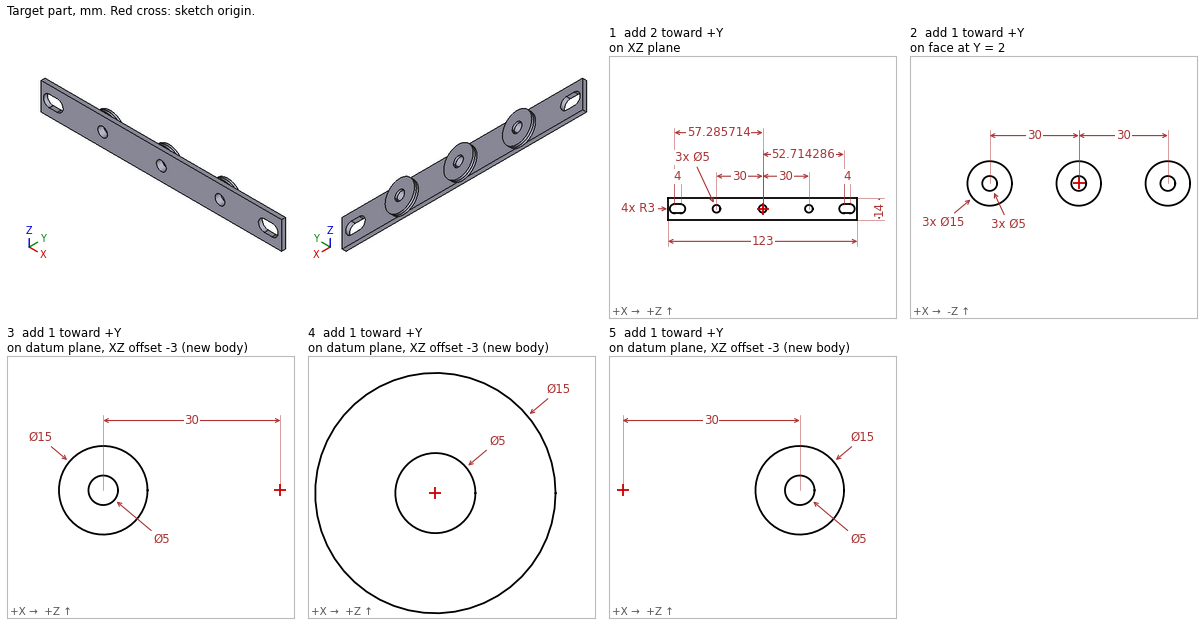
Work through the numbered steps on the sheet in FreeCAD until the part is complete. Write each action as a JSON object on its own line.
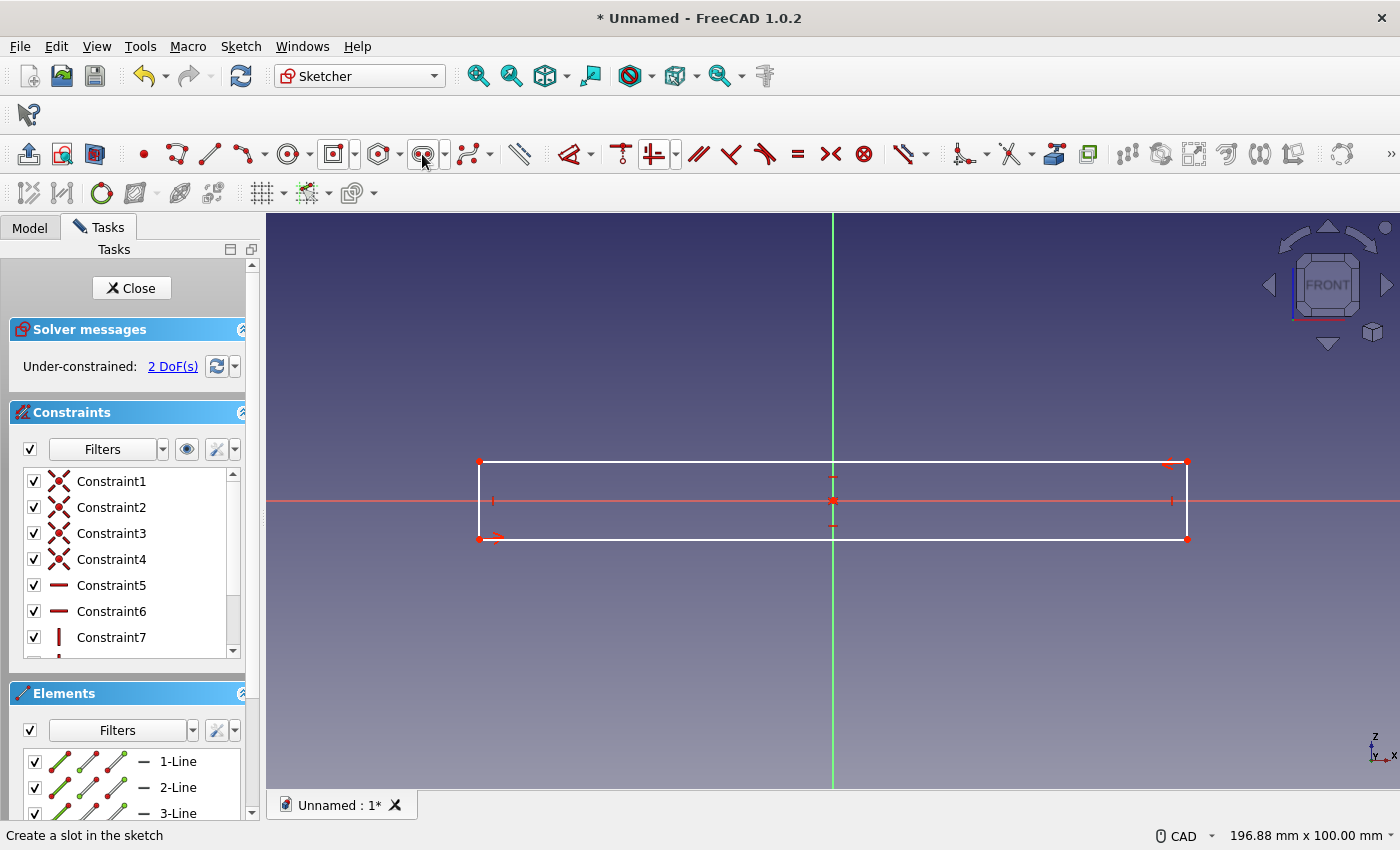
{"action": "scroll", "coordinate": [503, 501], "scroll_direction": "up", "scroll_amount": 2}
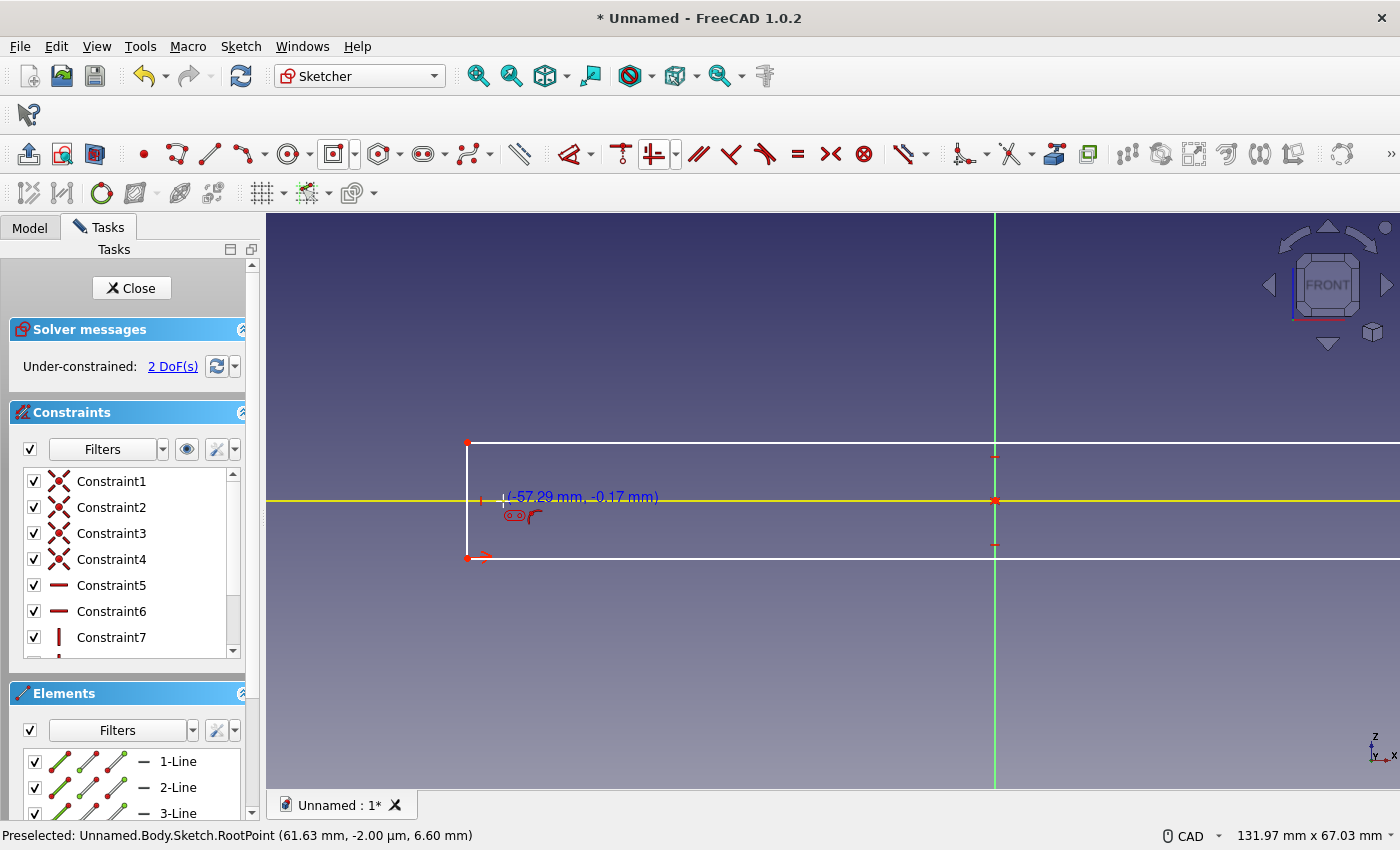
{"action": "left_click", "coordinate": [503, 501]}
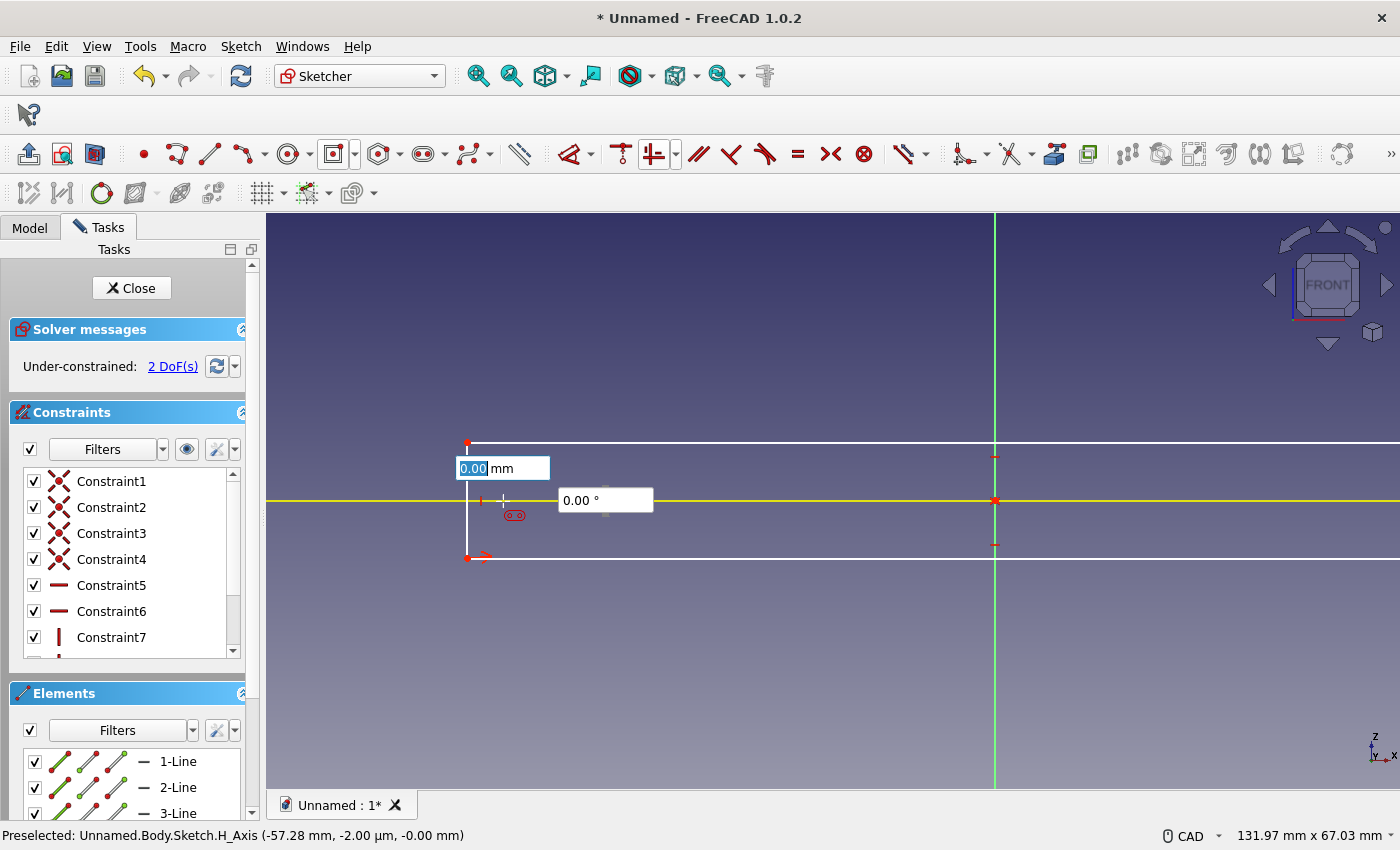
{"action": "left_click", "coordinate": [537, 492]}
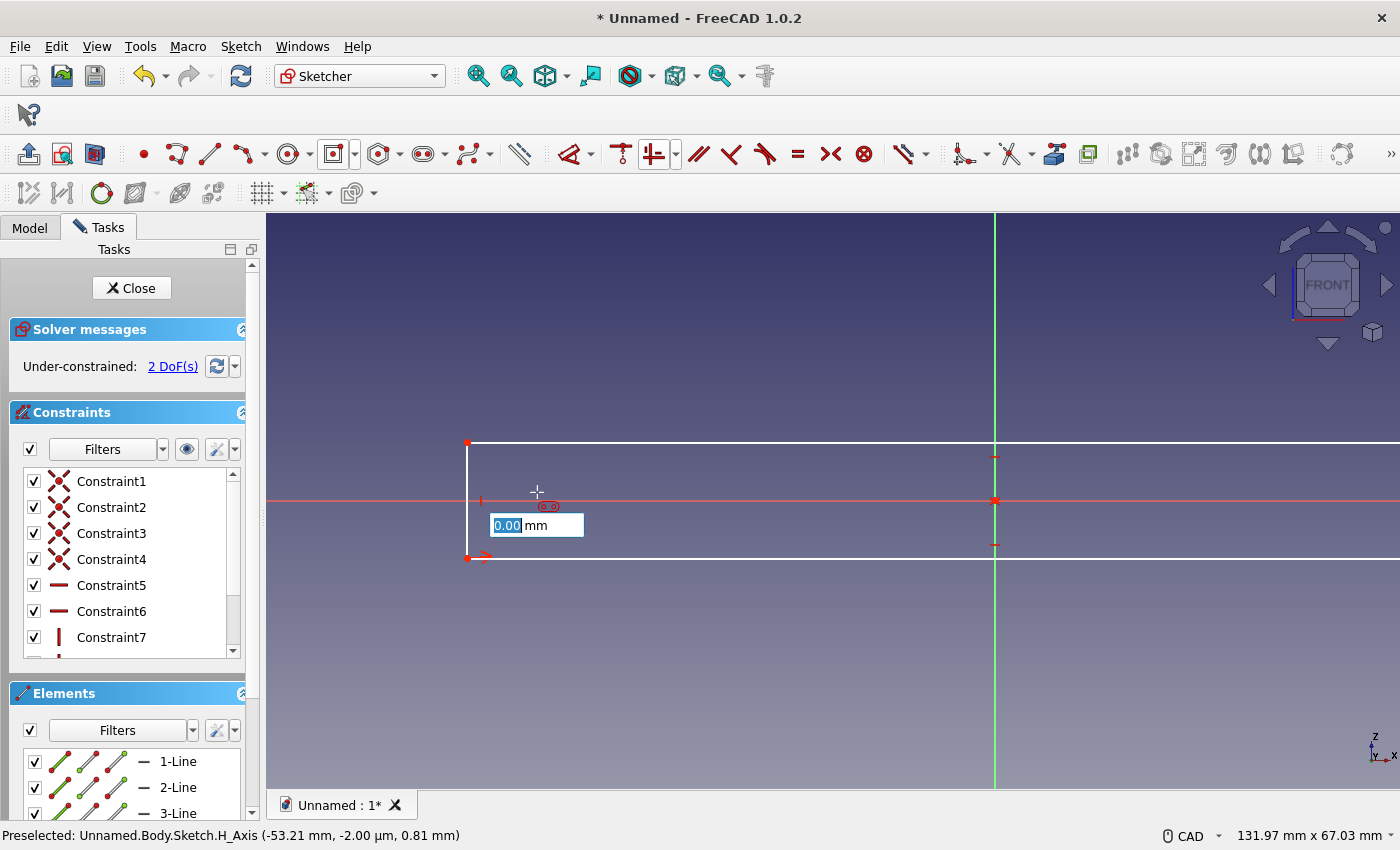
{"action": "left_click", "coordinate": [520, 527]}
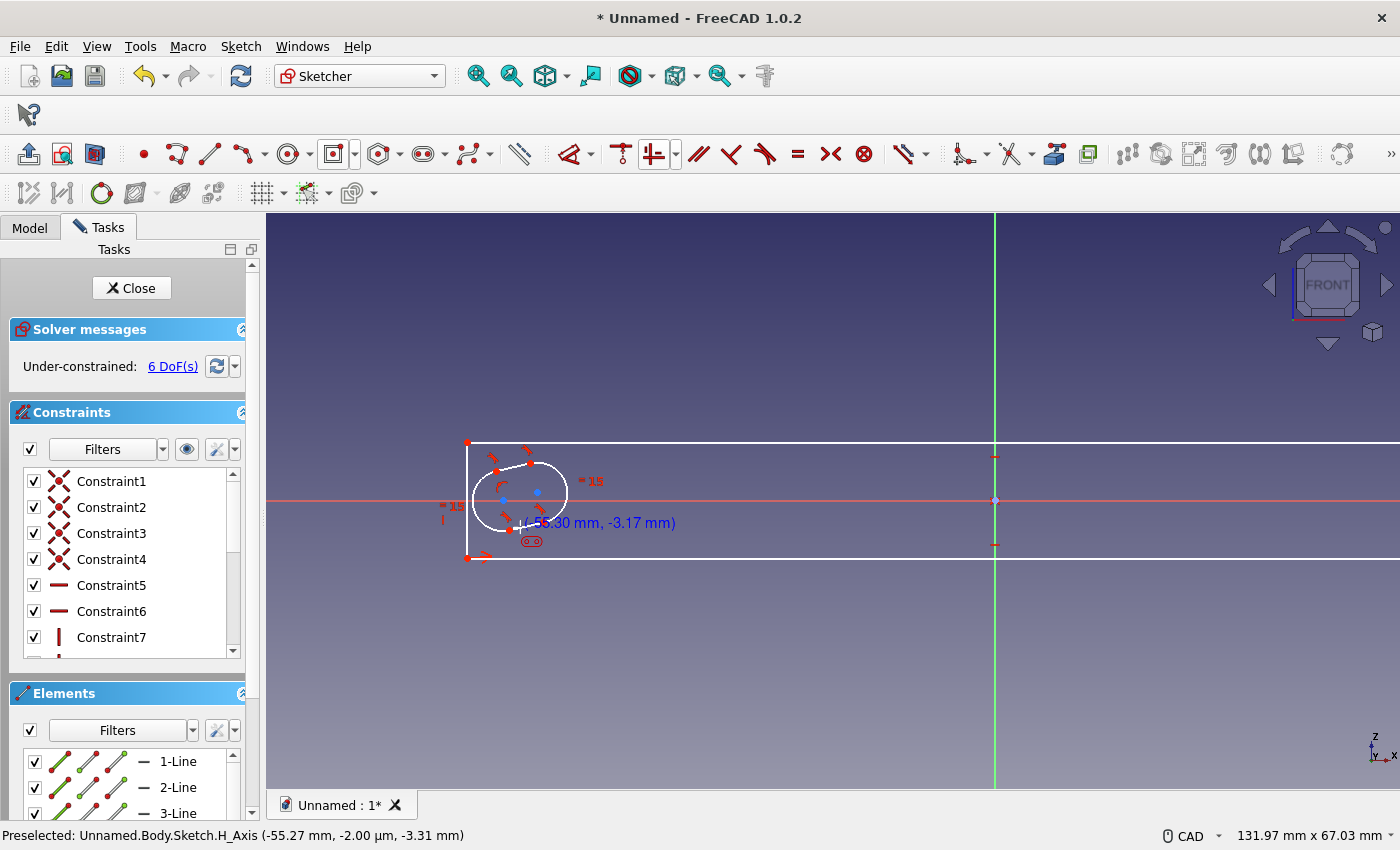
{"action": "scroll", "coordinate": [295, 502], "scroll_direction": "down", "scroll_amount": 2}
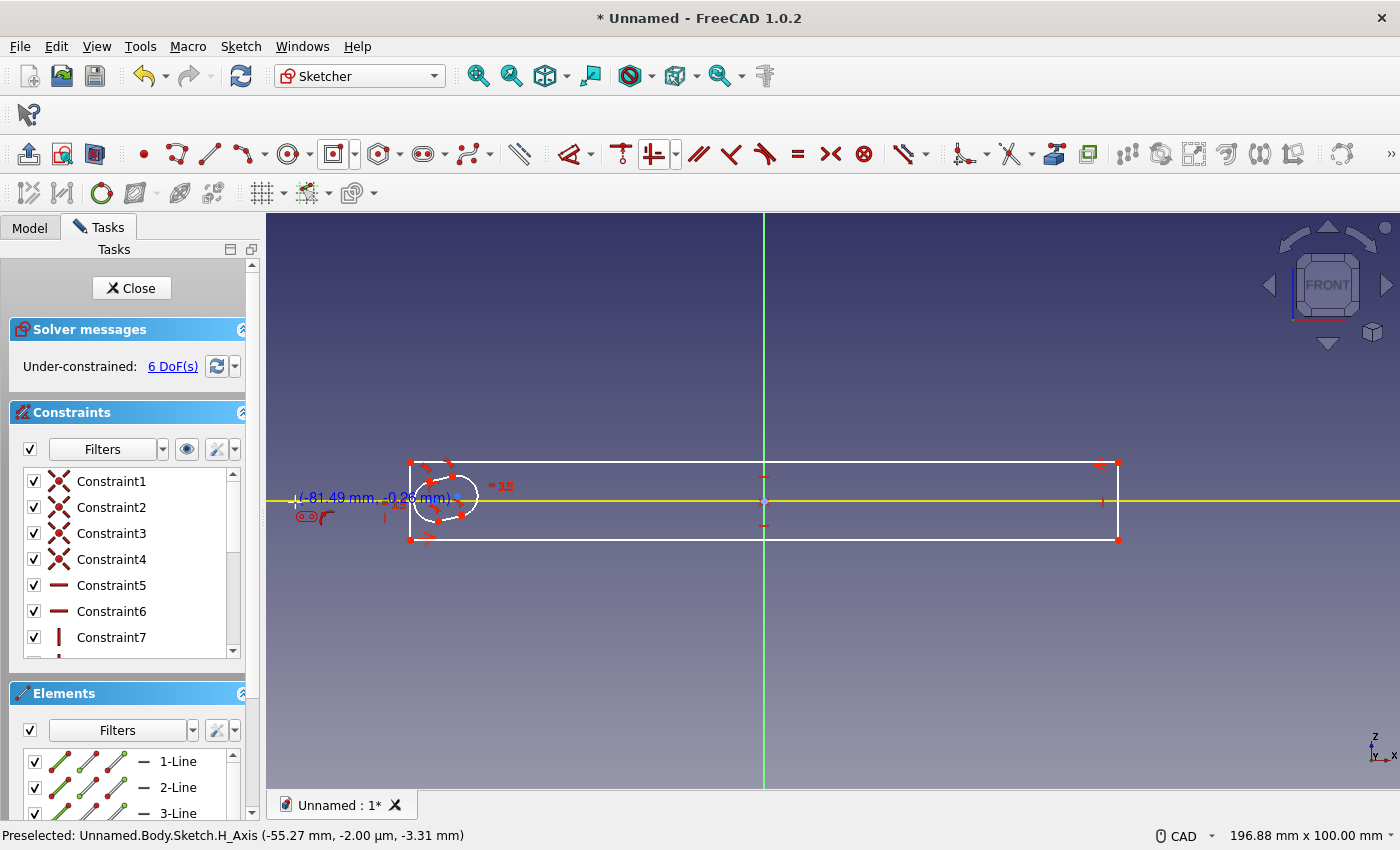
{"action": "scroll", "coordinate": [1068, 501], "scroll_direction": "up", "scroll_amount": 2}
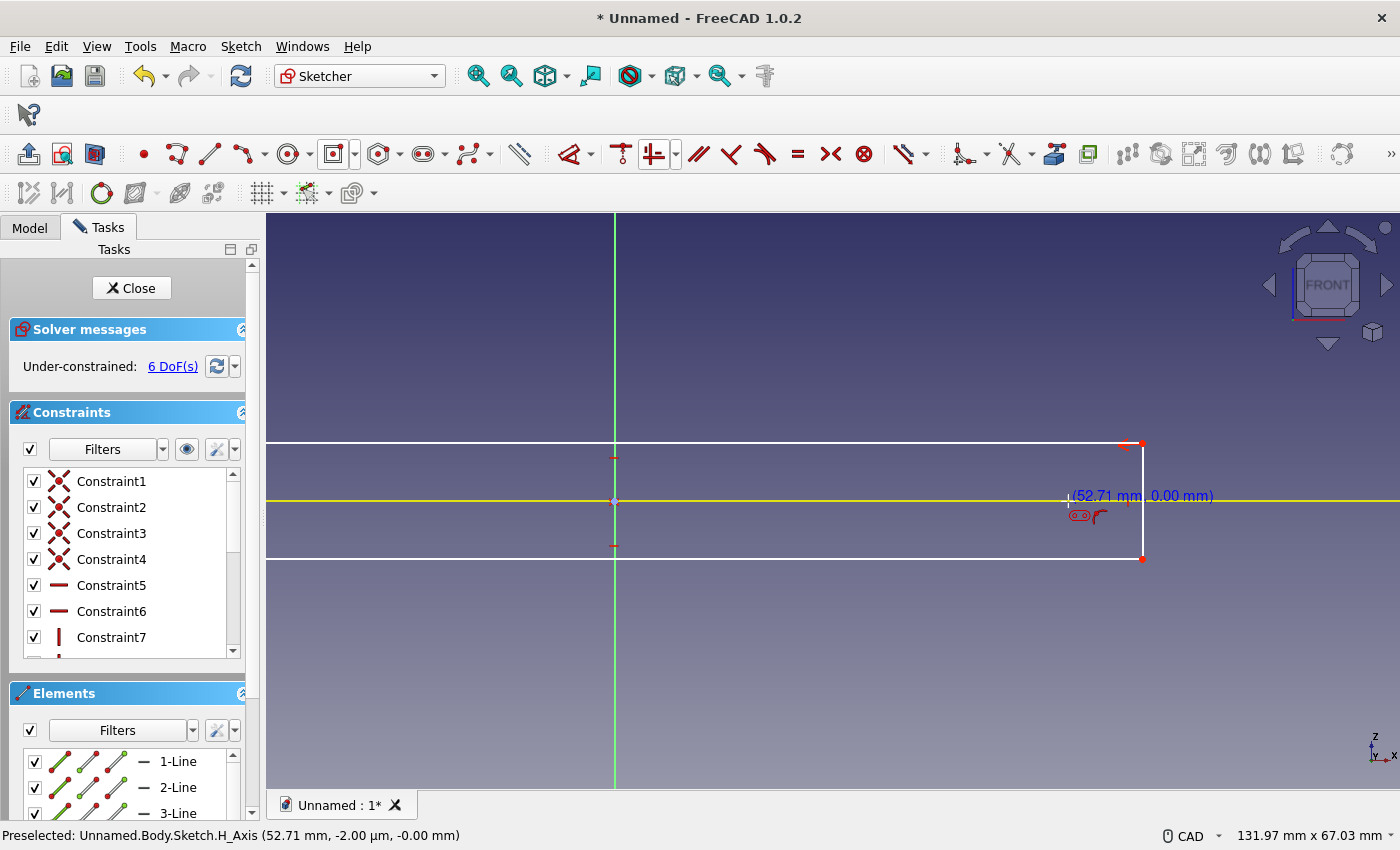
{"action": "left_click", "coordinate": [1068, 501]}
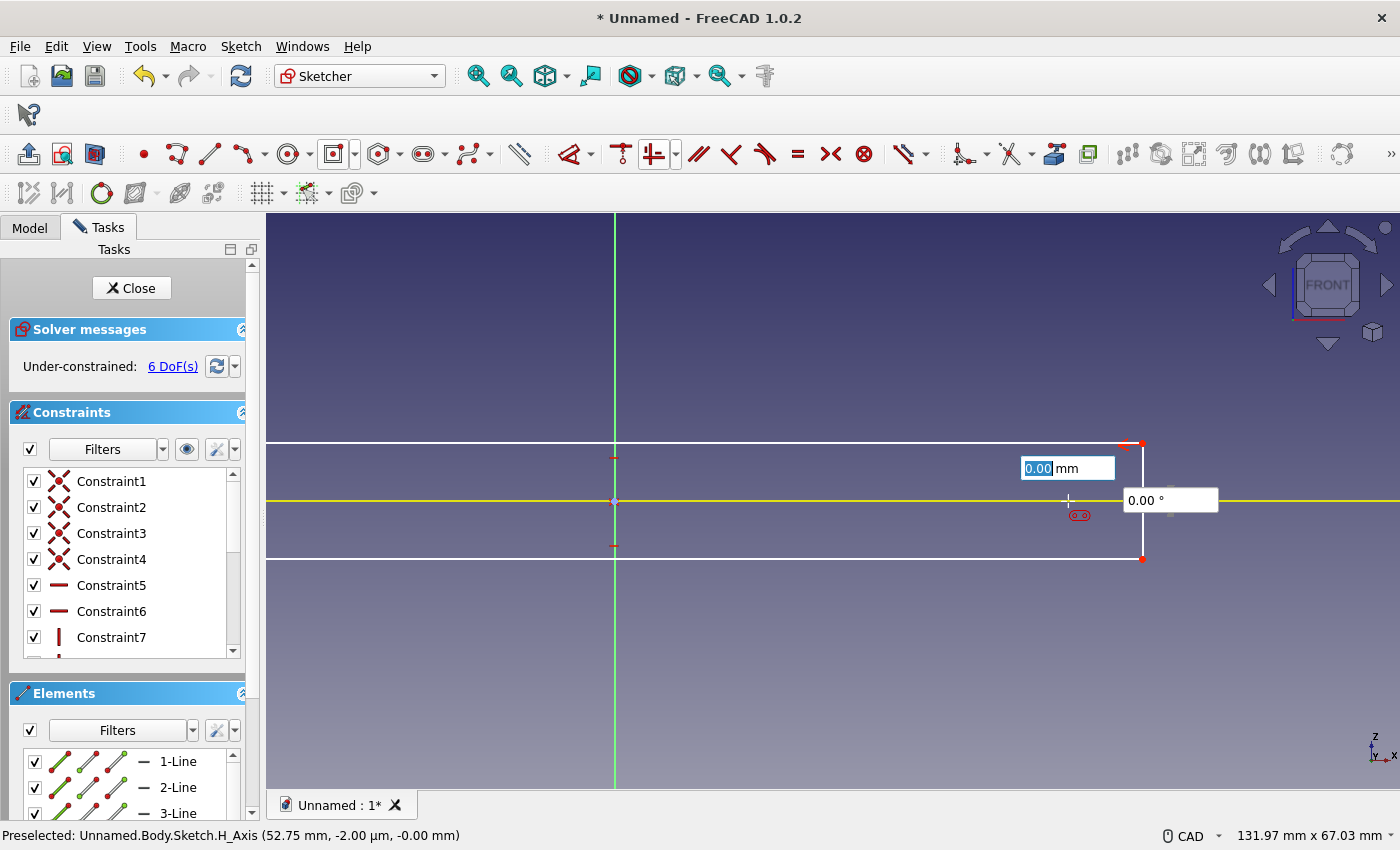
{"action": "left_click", "coordinate": [1102, 492]}